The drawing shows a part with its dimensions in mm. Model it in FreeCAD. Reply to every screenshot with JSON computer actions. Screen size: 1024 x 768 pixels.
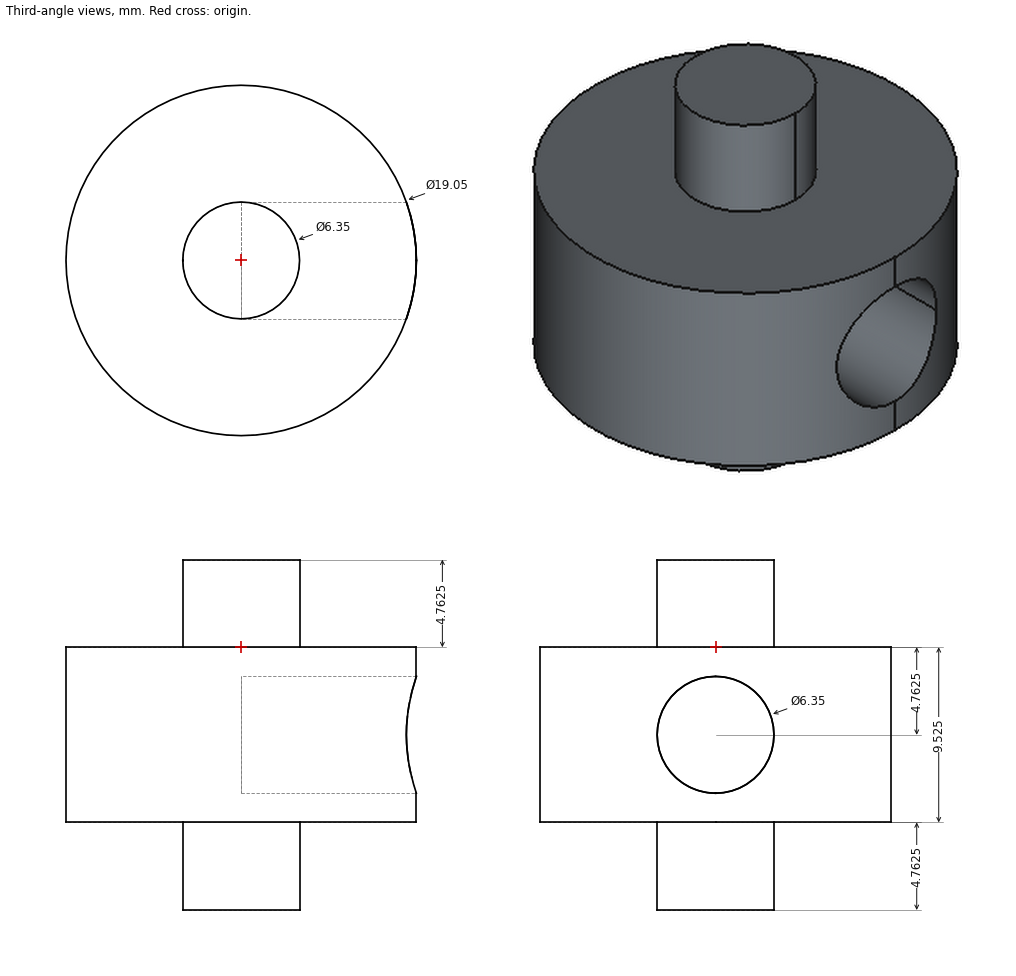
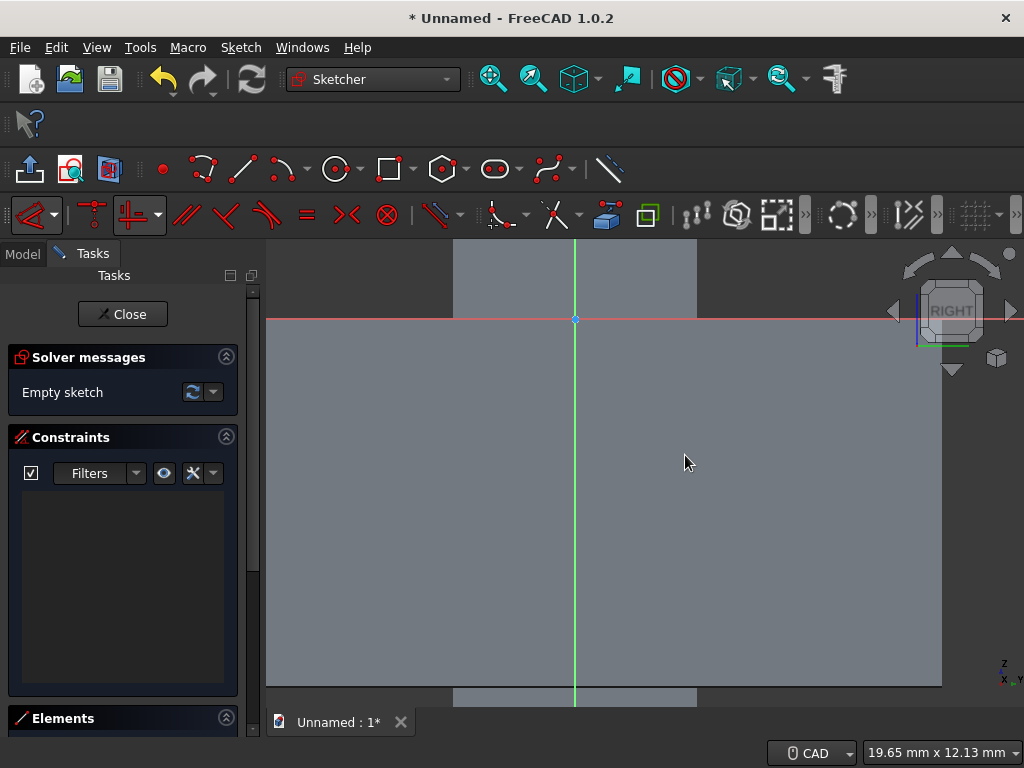
{"action": "left_click", "coordinate": [336, 170]}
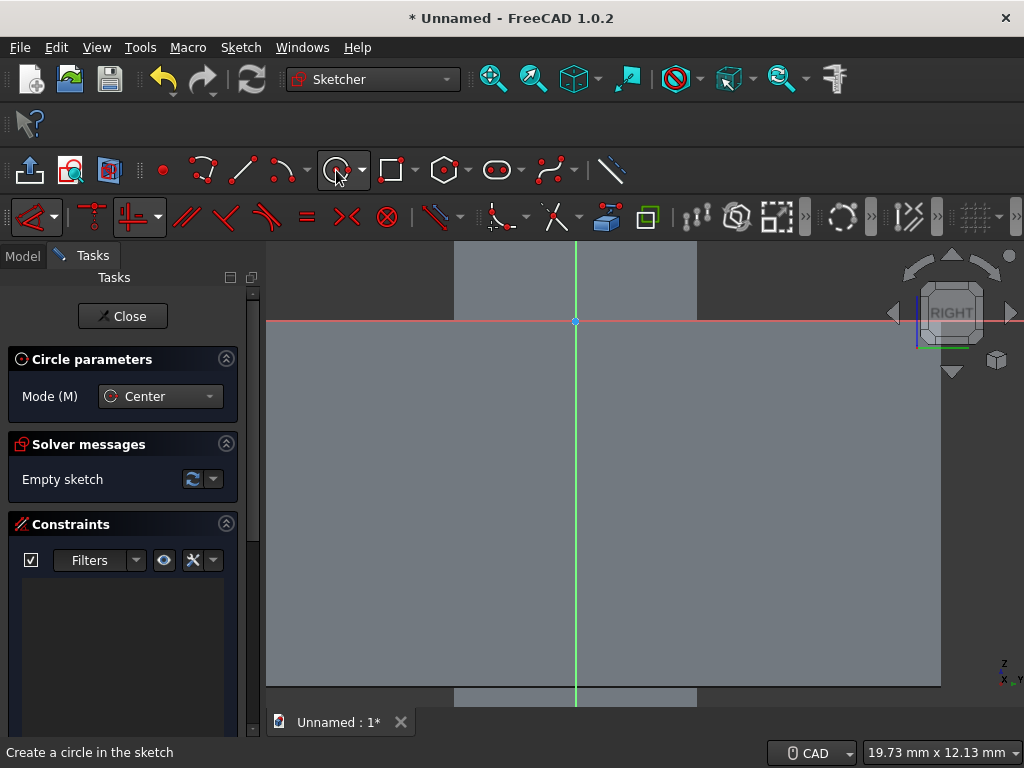
{"action": "left_click", "coordinate": [576, 504]}
{"action": "left_click", "coordinate": [662, 418]}
{"action": "key", "text": "Escape"}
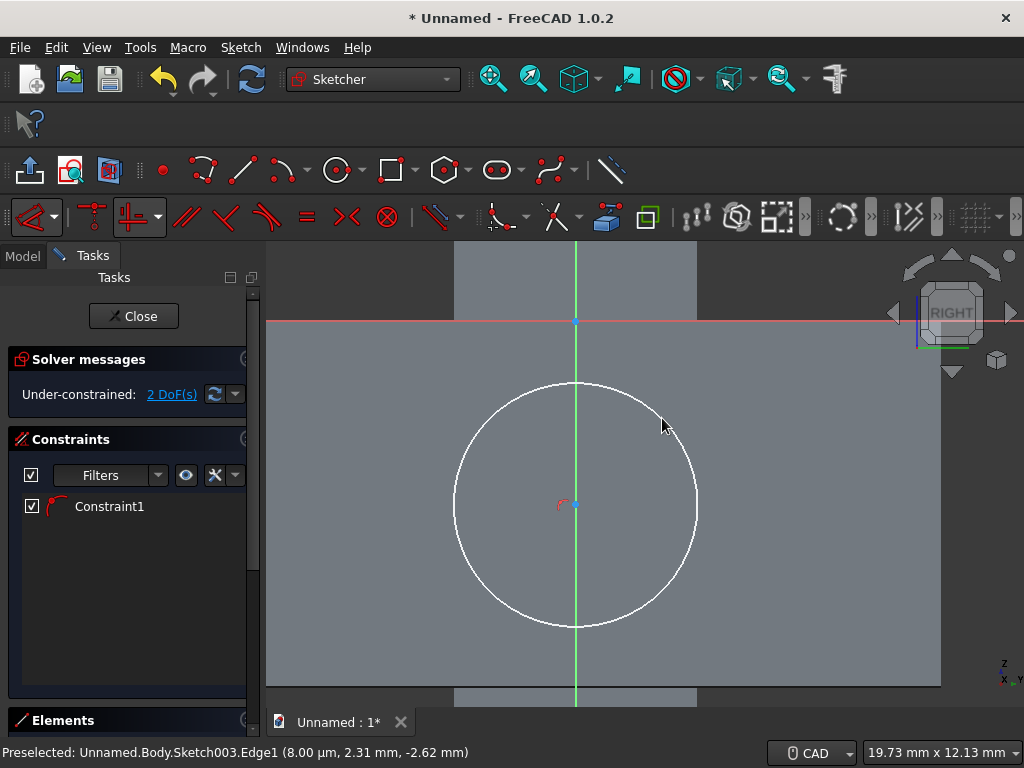
{"action": "left_click", "coordinate": [662, 419]}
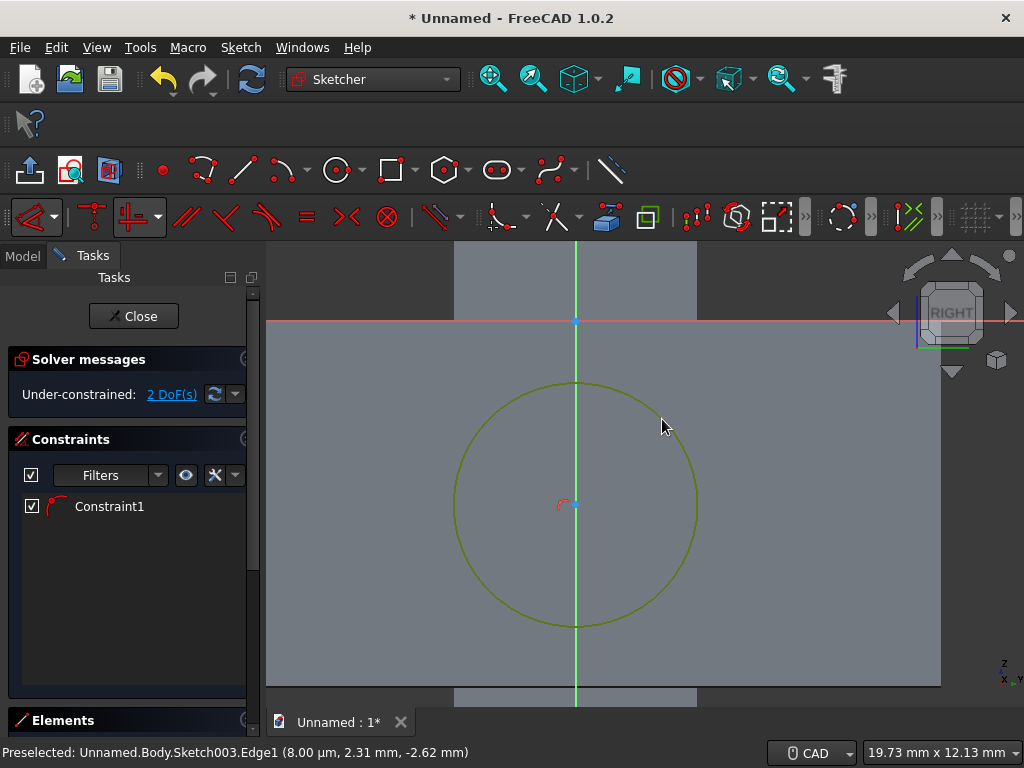
{"action": "key", "text": "k o"}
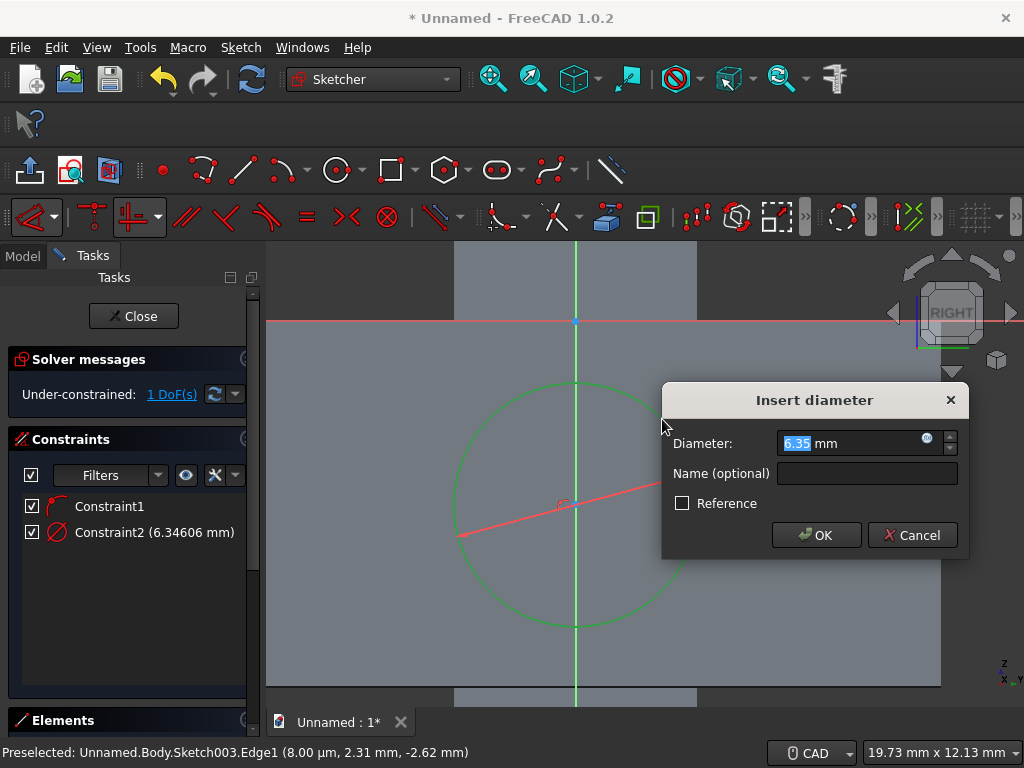
{"action": "type", "text": "6.35"}
{"action": "key", "text": "Return"}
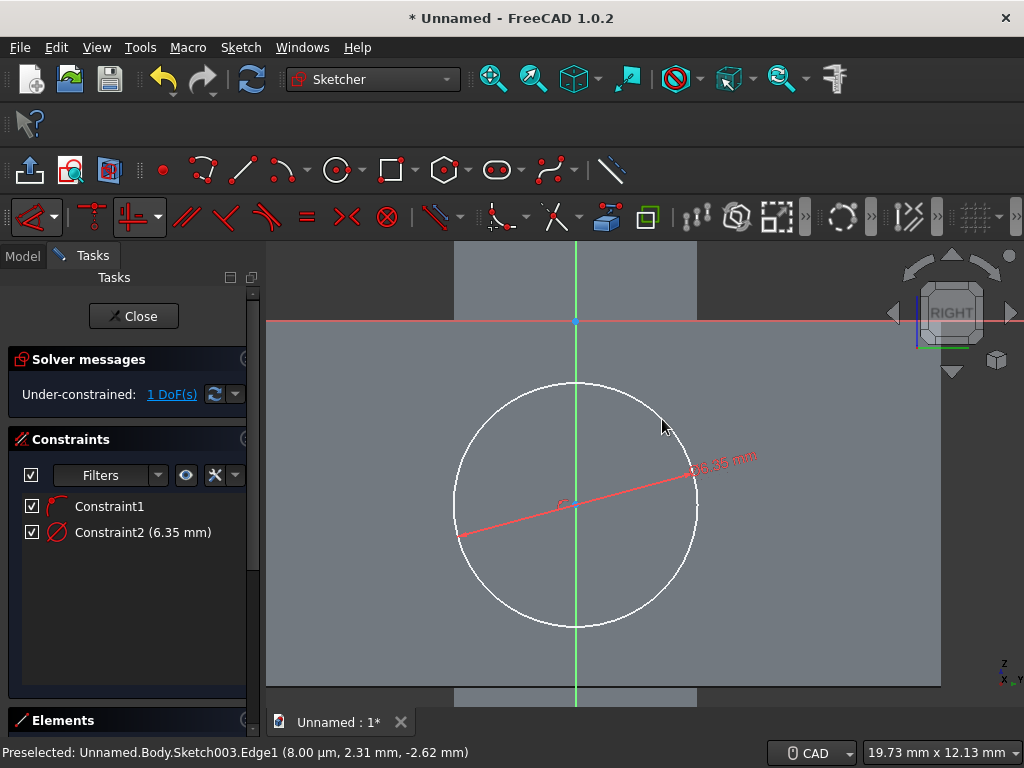
{"action": "left_click", "coordinate": [576, 505]}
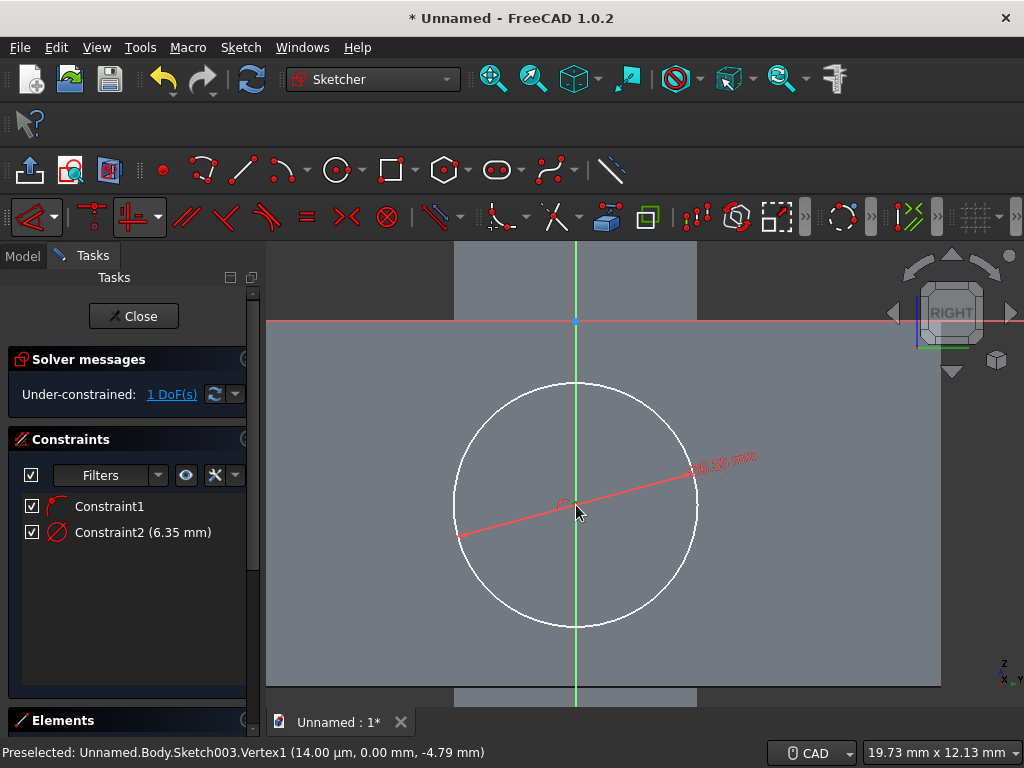
{"action": "key", "text": "i"}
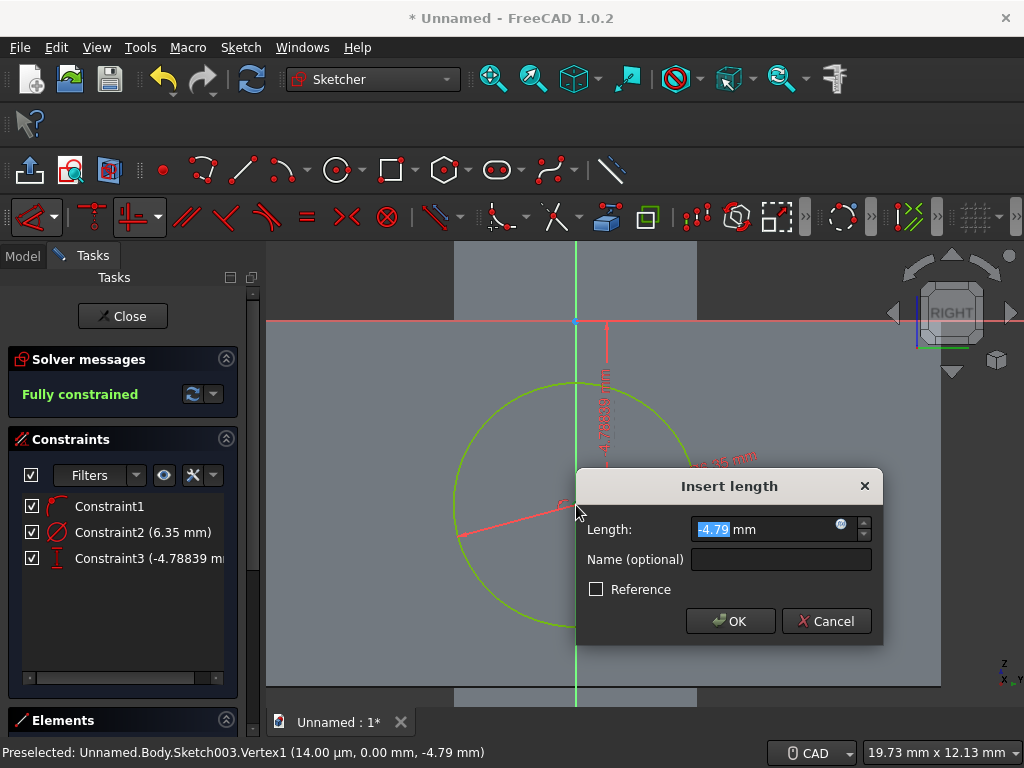
{"action": "type", "text": "-4.7625"}
{"action": "key", "text": "Return"}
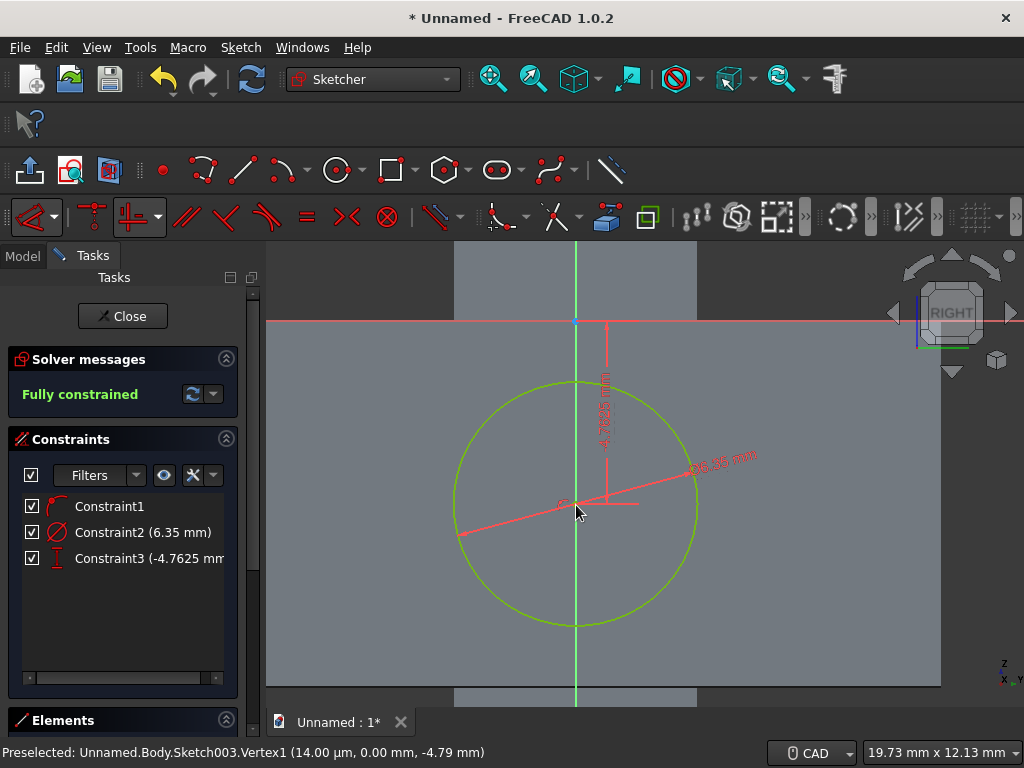
{"action": "left_click", "coordinate": [123, 316]}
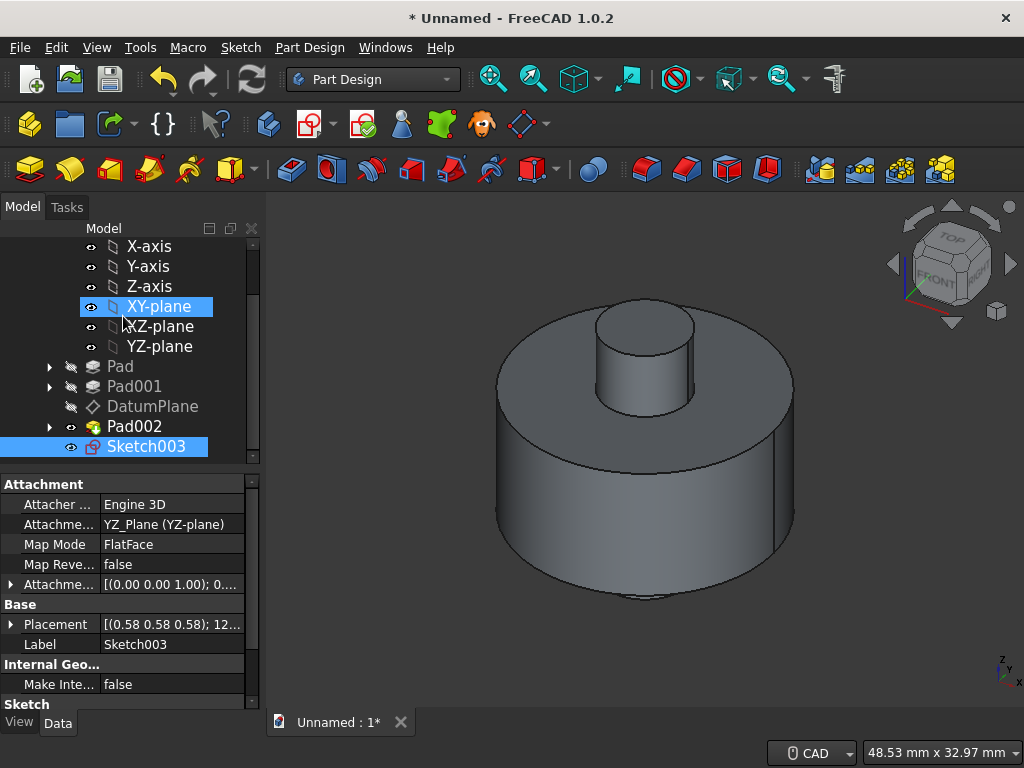
{"action": "left_click", "coordinate": [292, 170]}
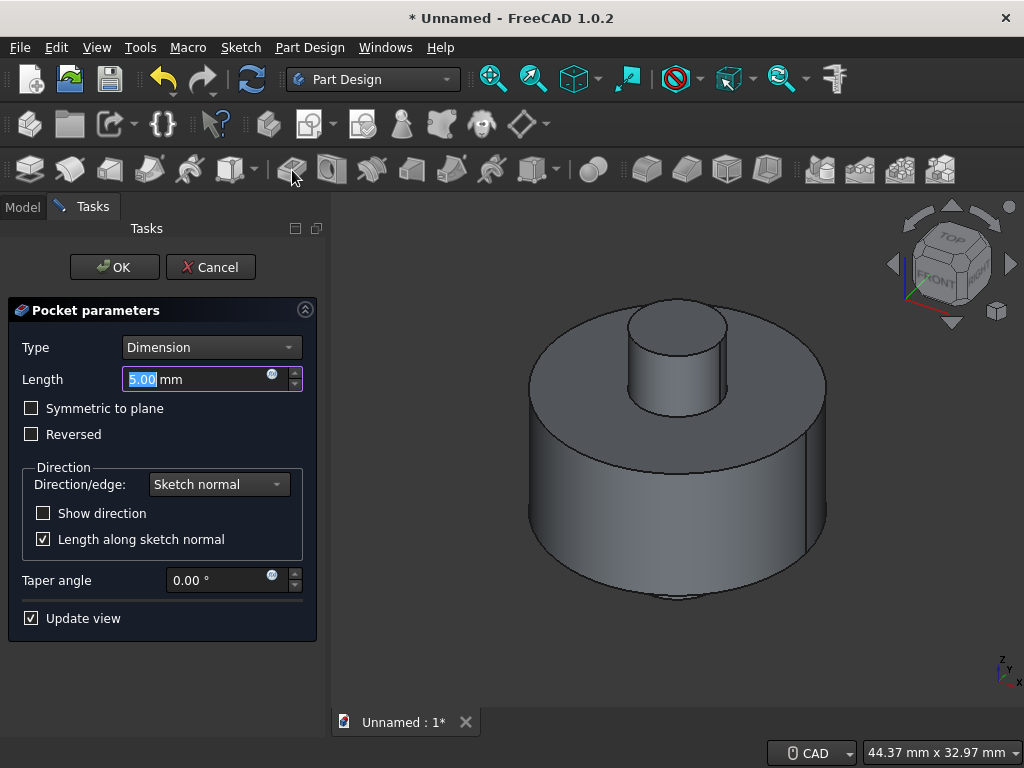
{"action": "left_click", "coordinate": [212, 348]}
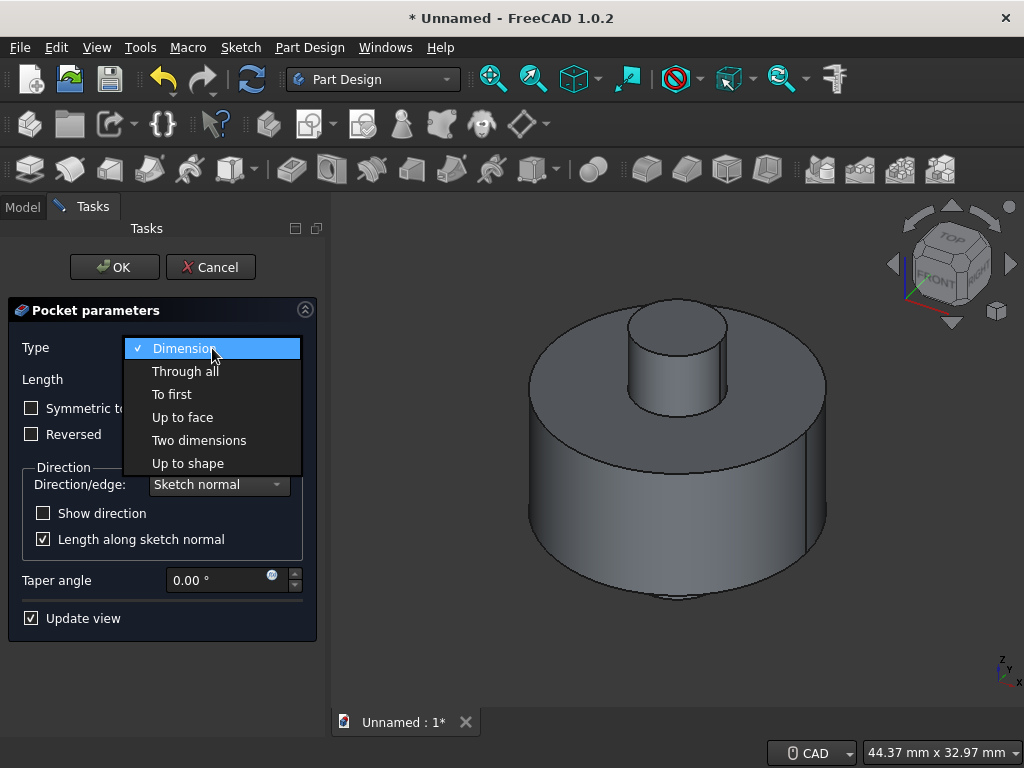
{"action": "left_click", "coordinate": [212, 372]}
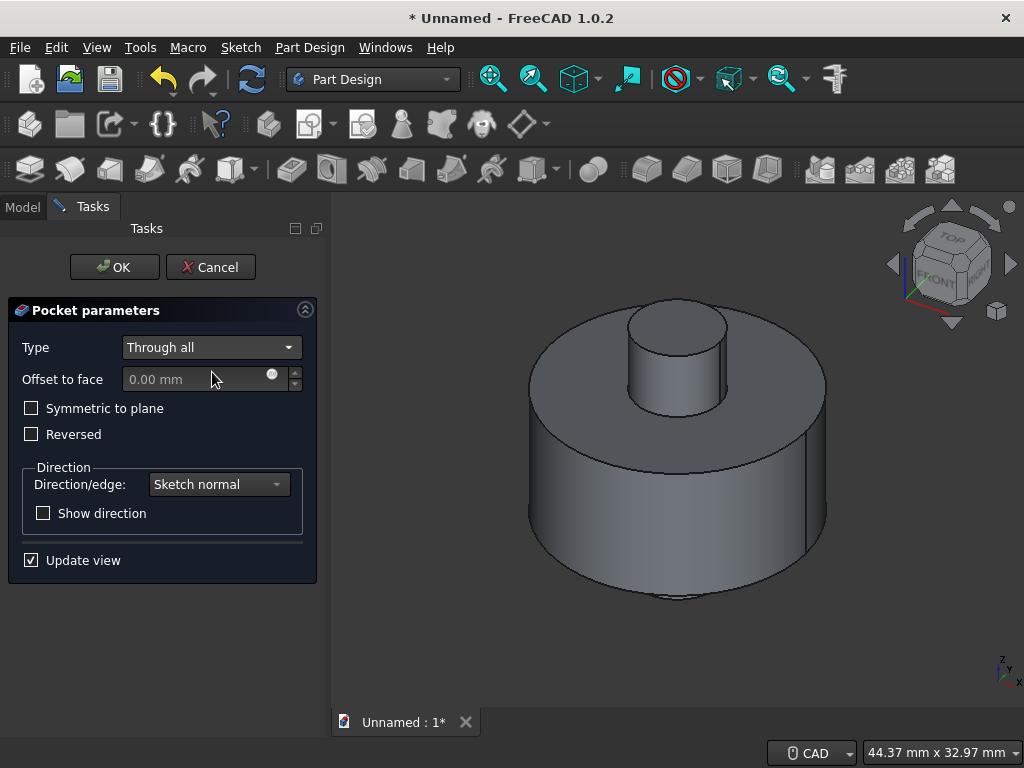
{"action": "left_click", "coordinate": [30, 434]}